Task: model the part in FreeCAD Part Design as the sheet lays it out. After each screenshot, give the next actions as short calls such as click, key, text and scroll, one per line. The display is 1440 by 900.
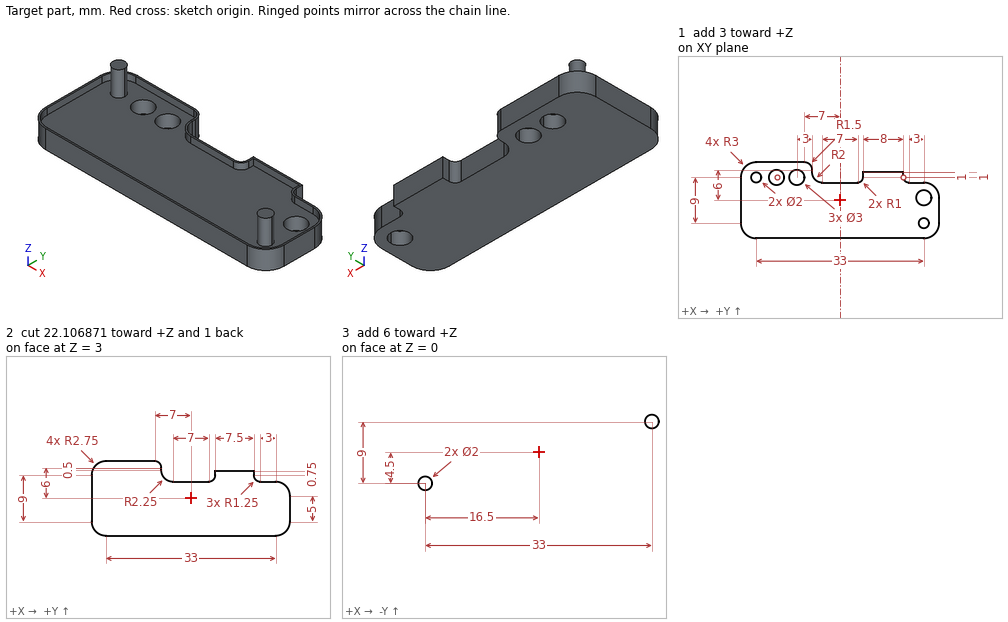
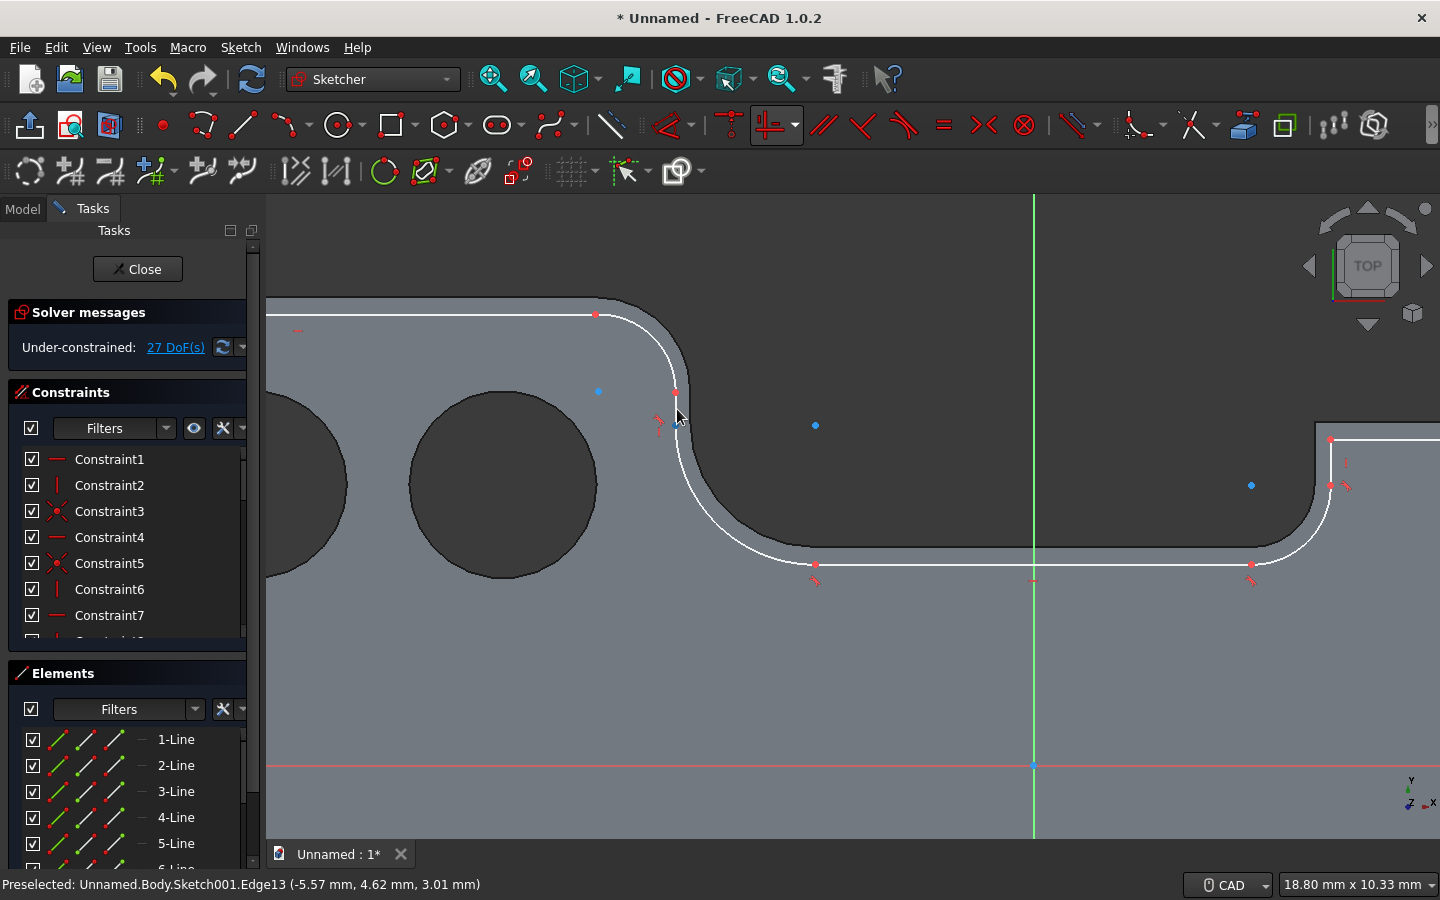
click(676, 409)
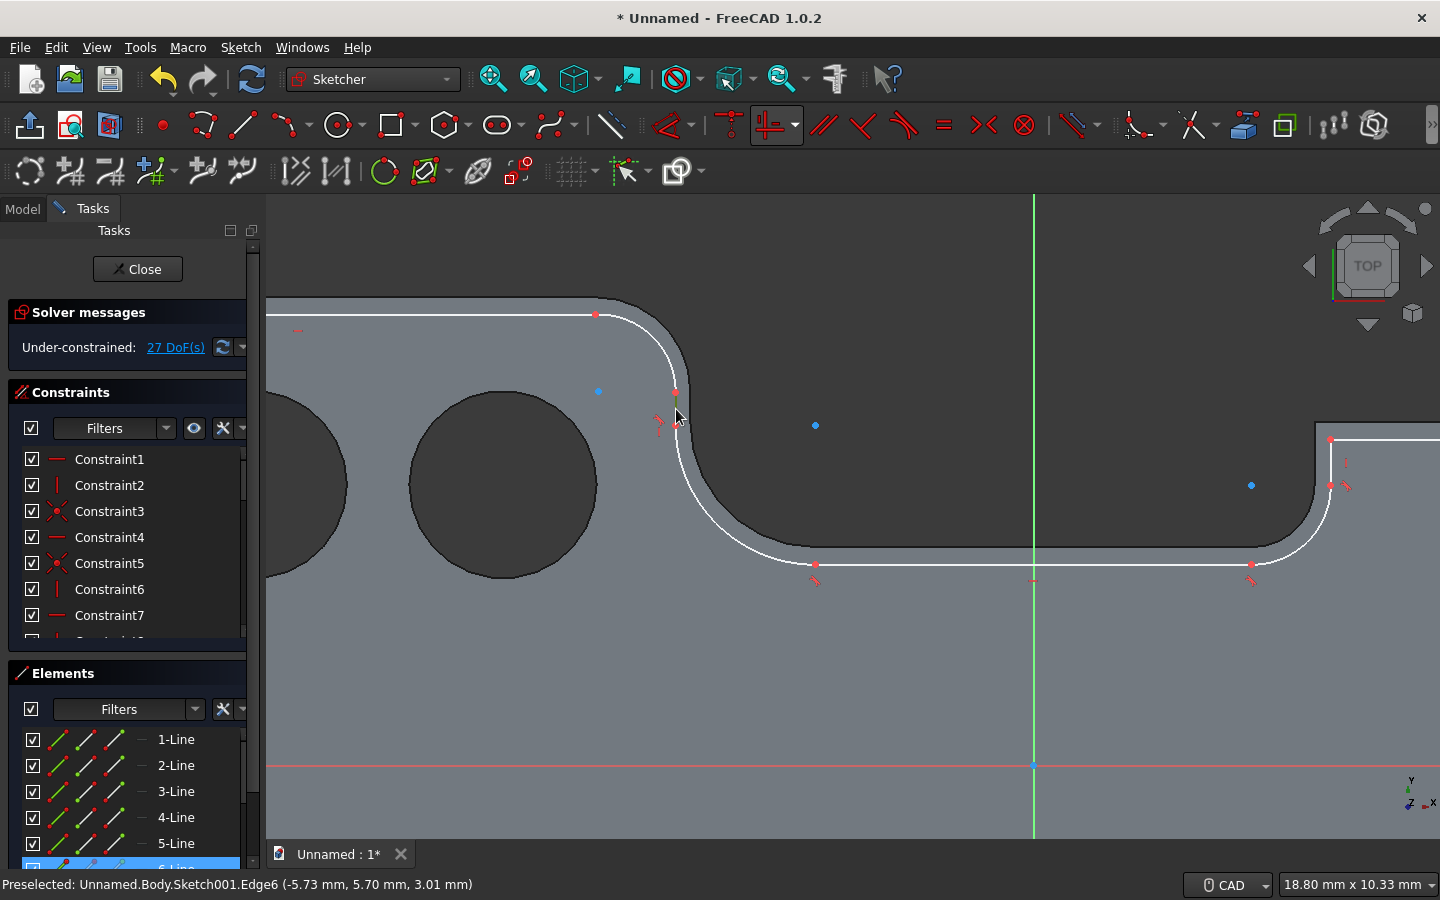
click(667, 357)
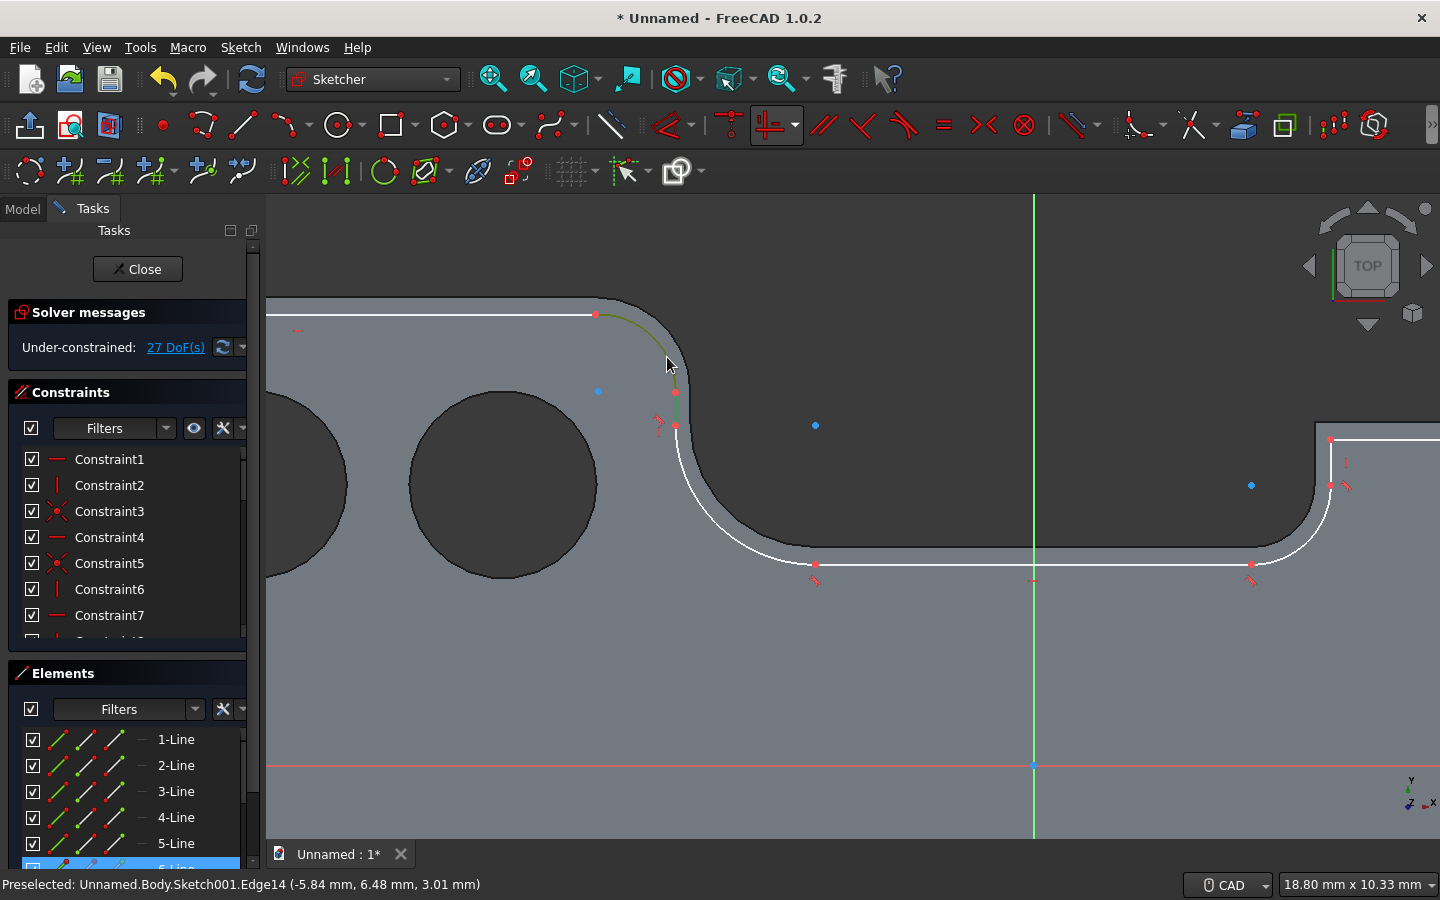
click(904, 126)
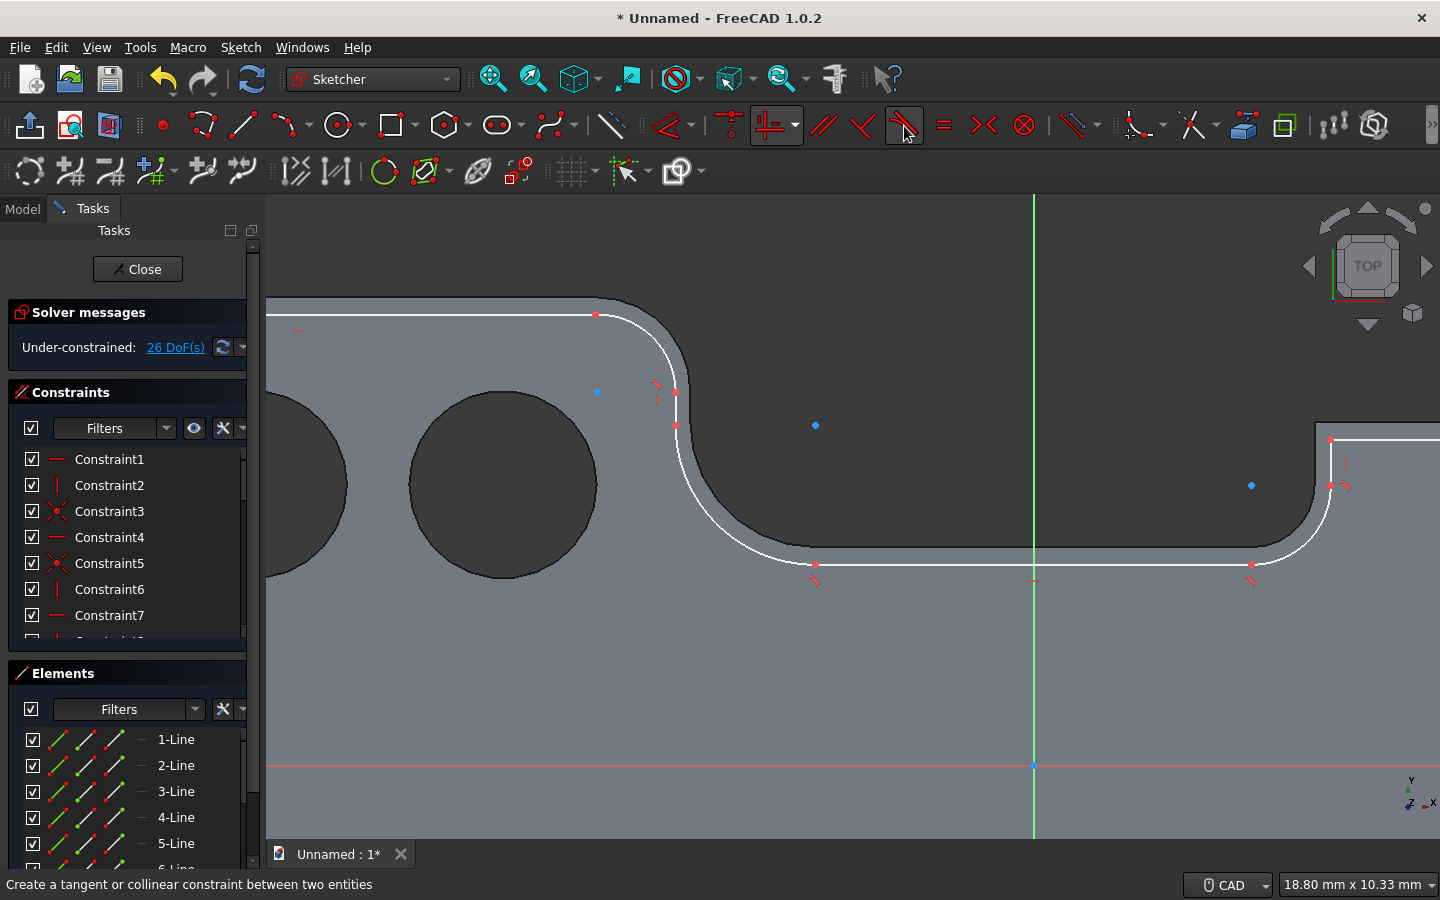
scroll(677, 409, down, 6)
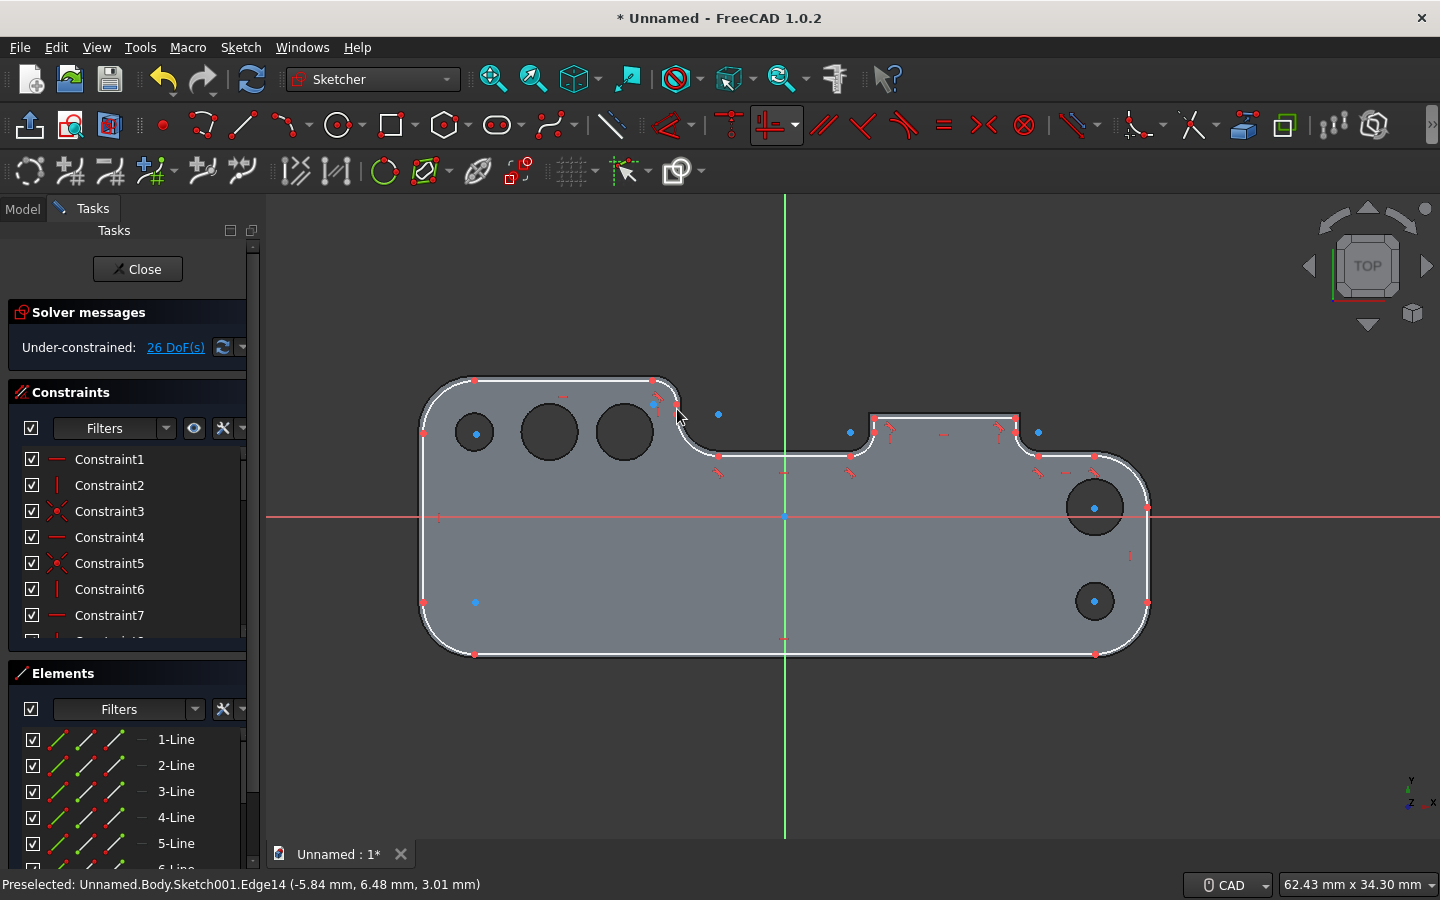
click(599, 381)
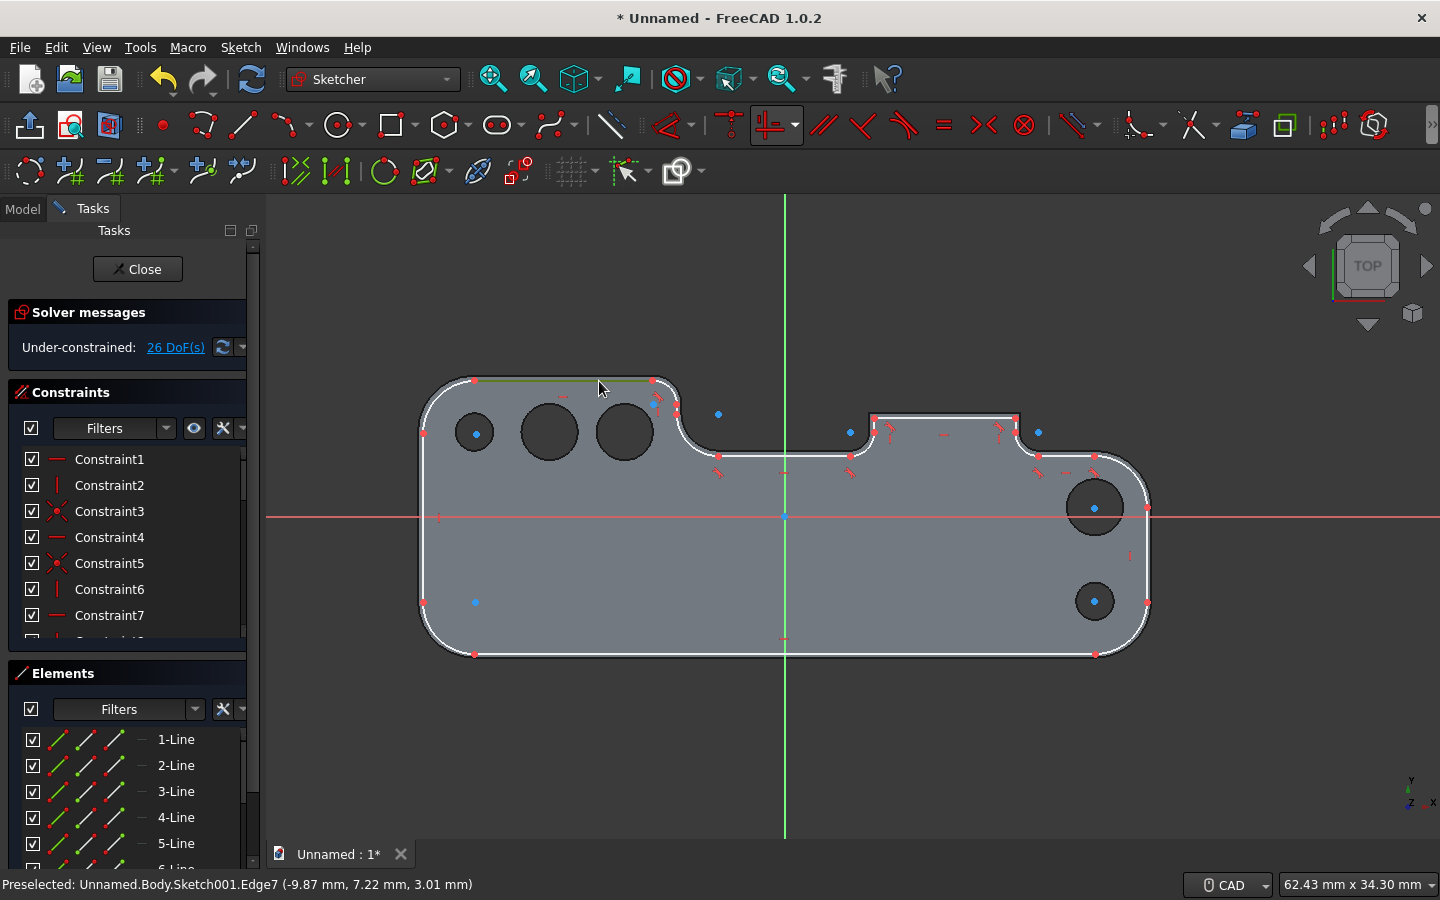
scroll(674, 394, up, 2)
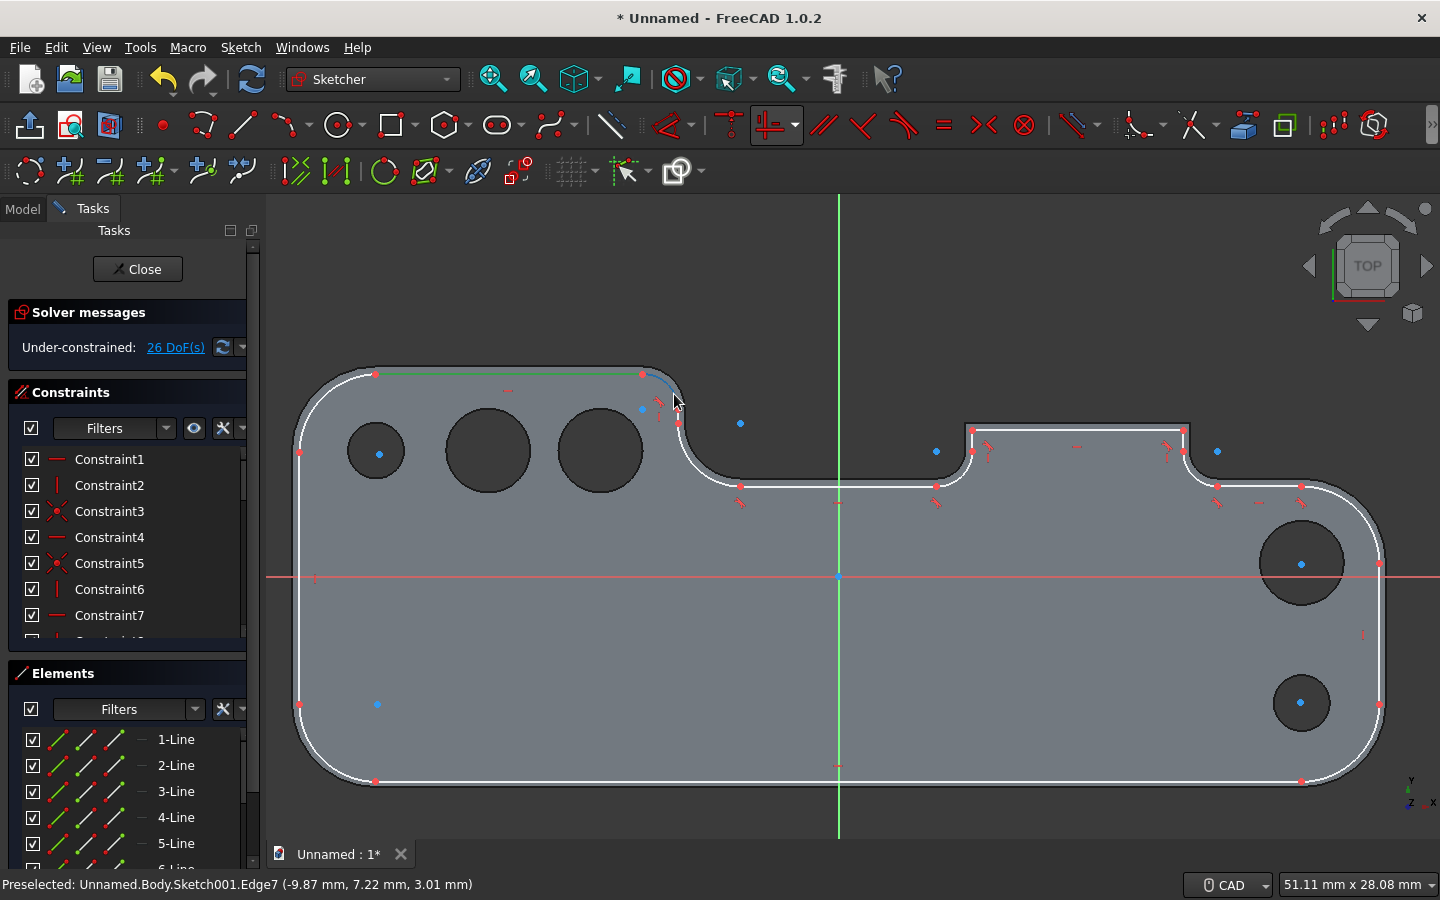
click(674, 393)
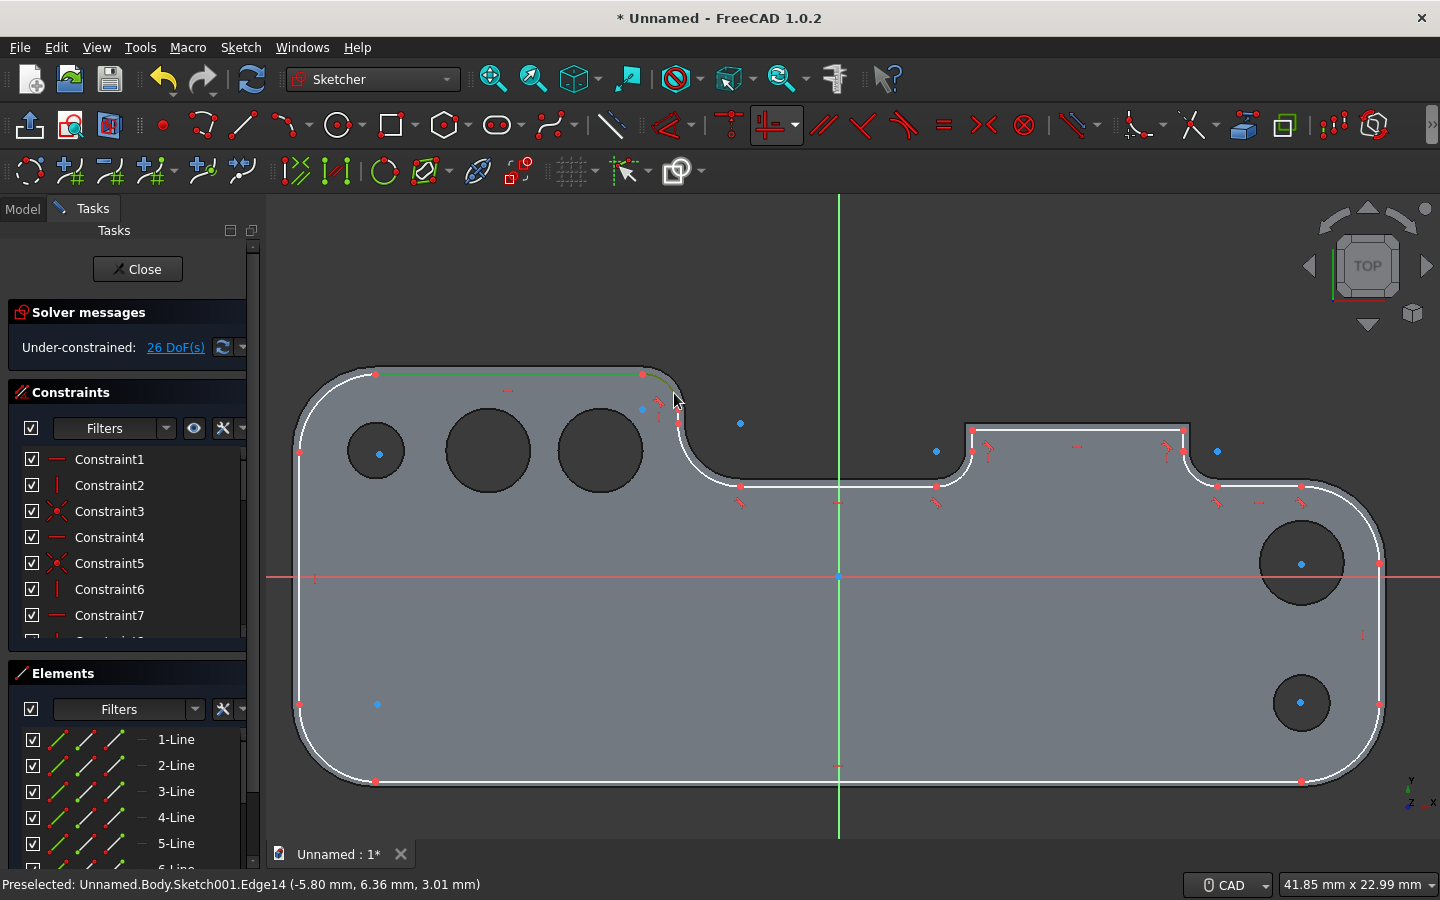
click(904, 126)